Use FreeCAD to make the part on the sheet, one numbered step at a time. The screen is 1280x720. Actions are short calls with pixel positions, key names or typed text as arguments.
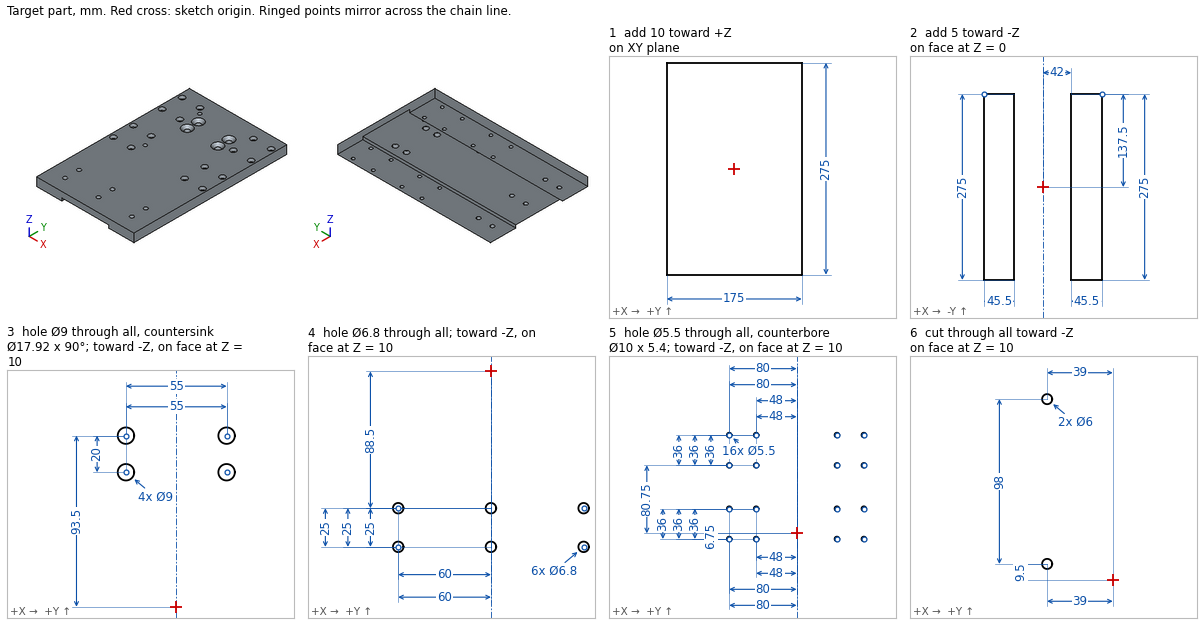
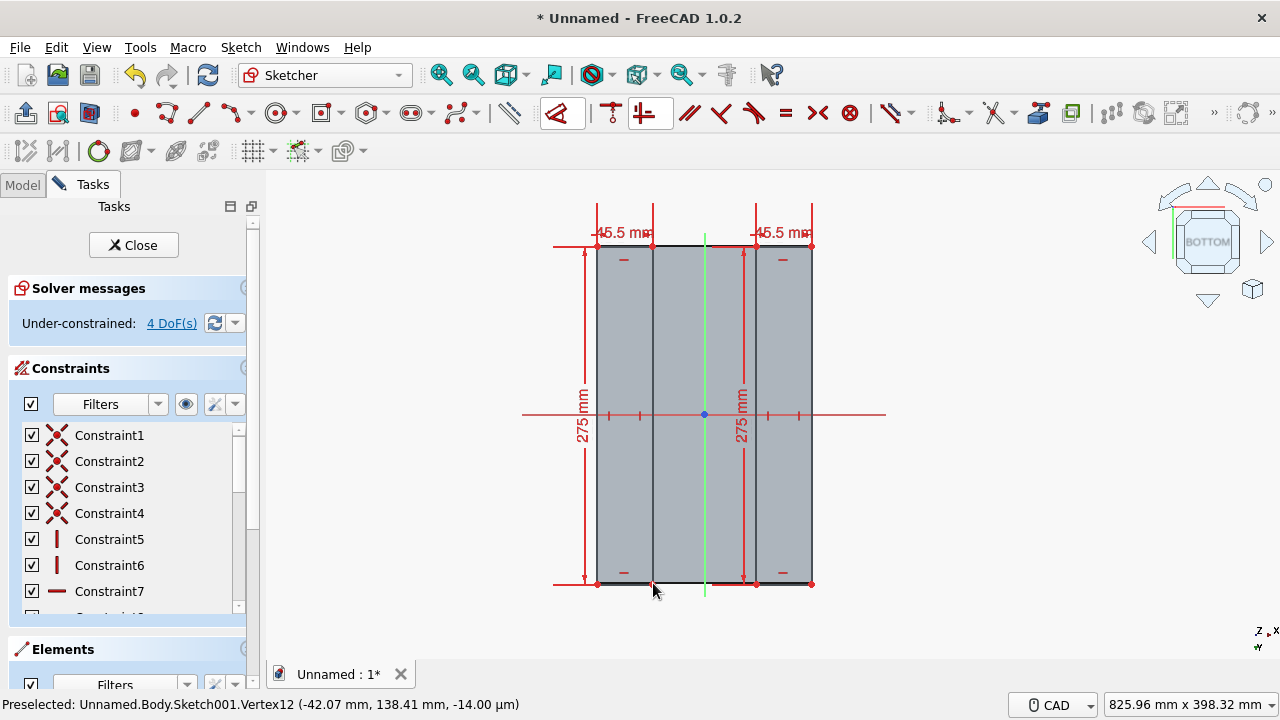
click(812, 247)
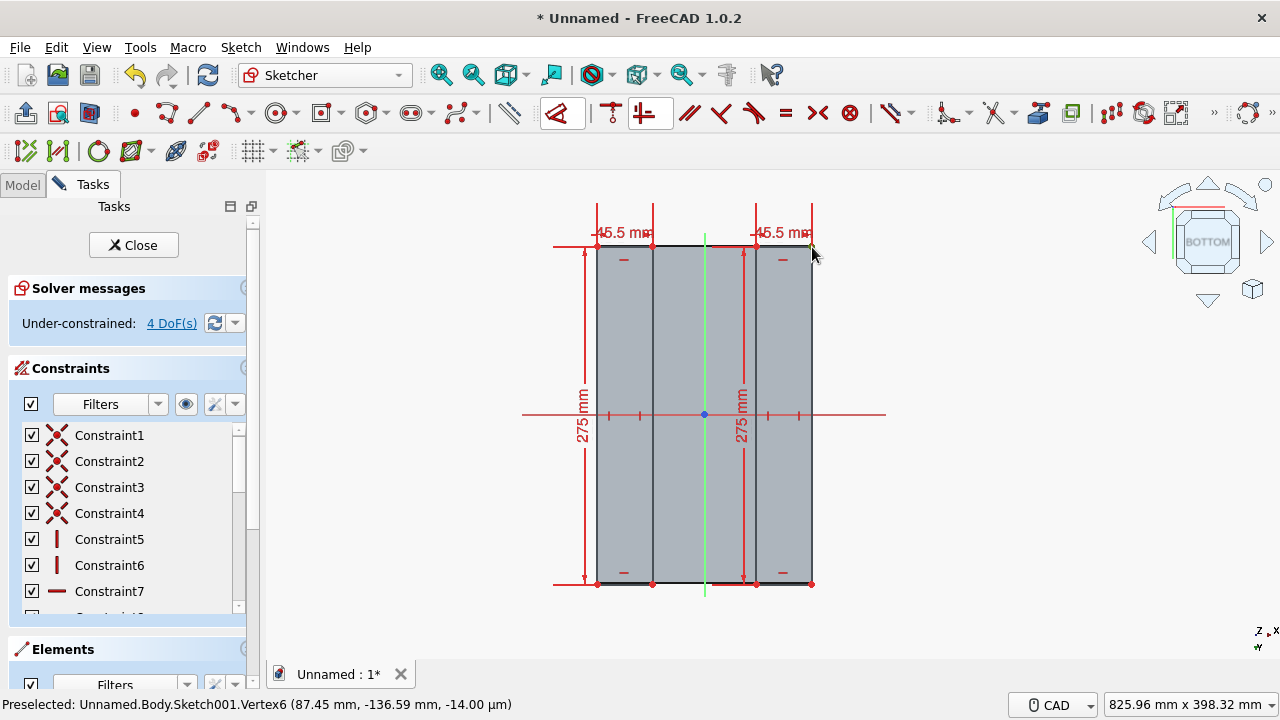
click(597, 247)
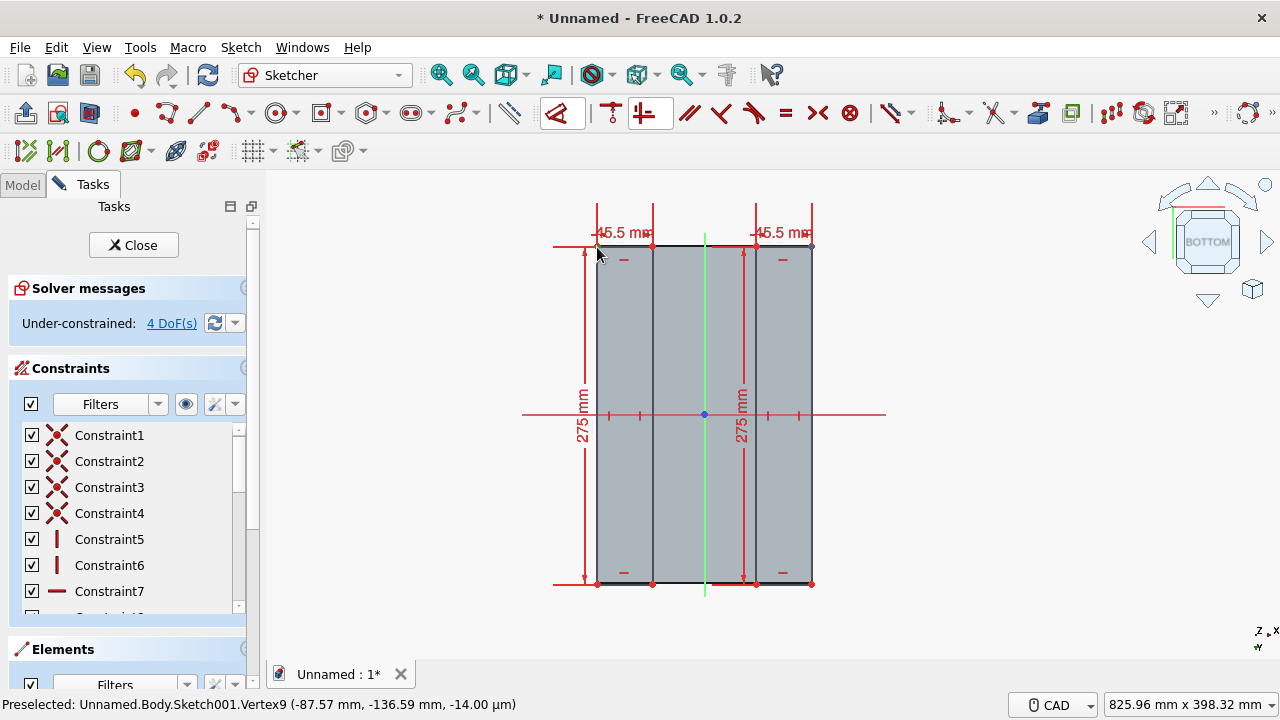
click(705, 600)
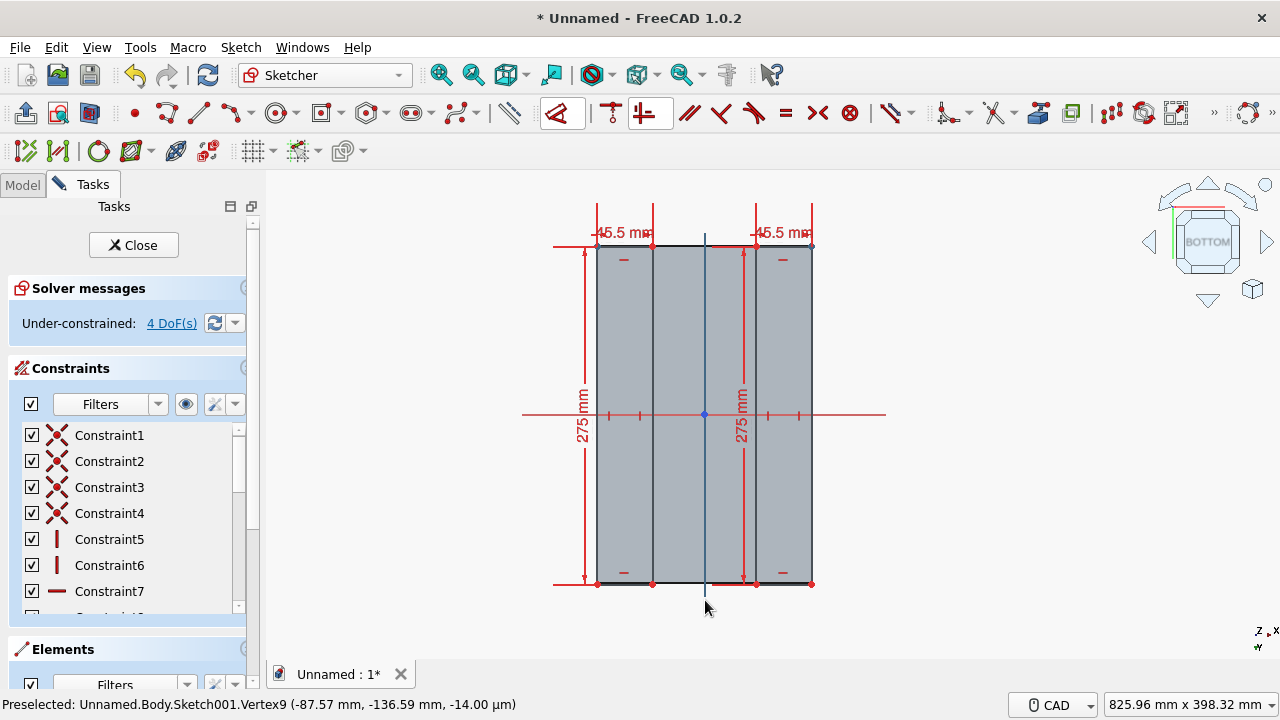
key(s)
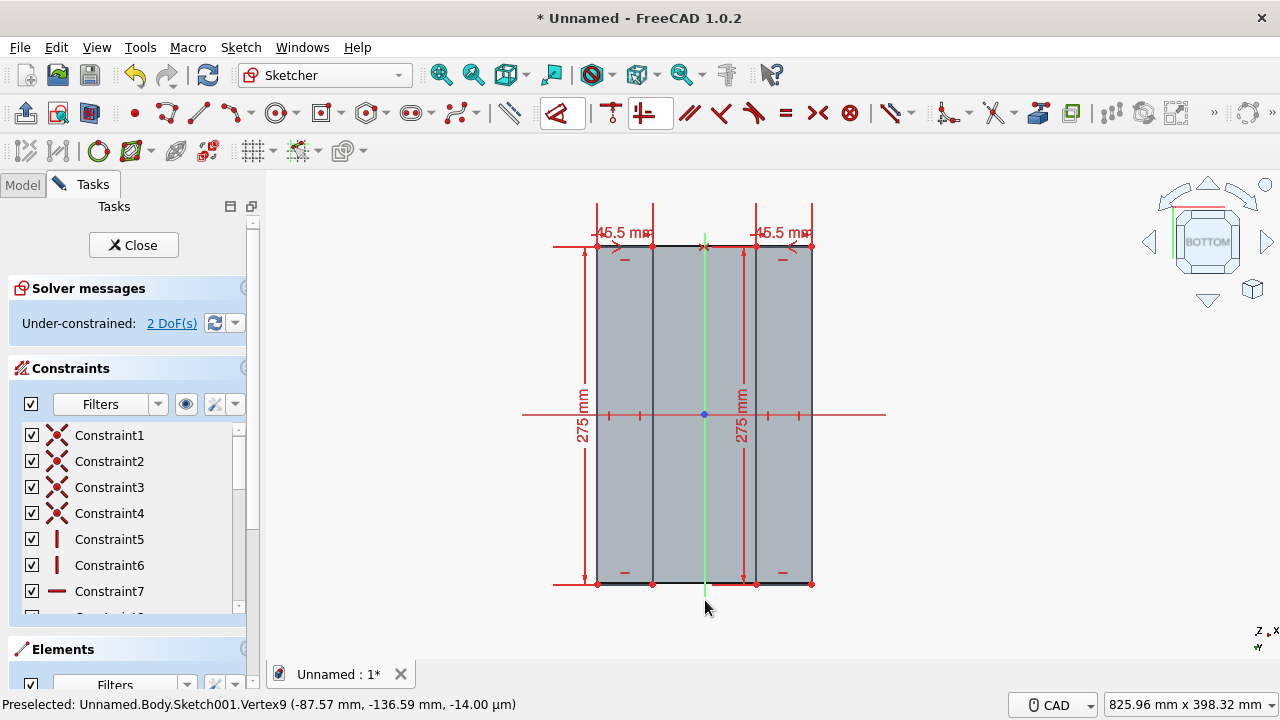
click(556, 114)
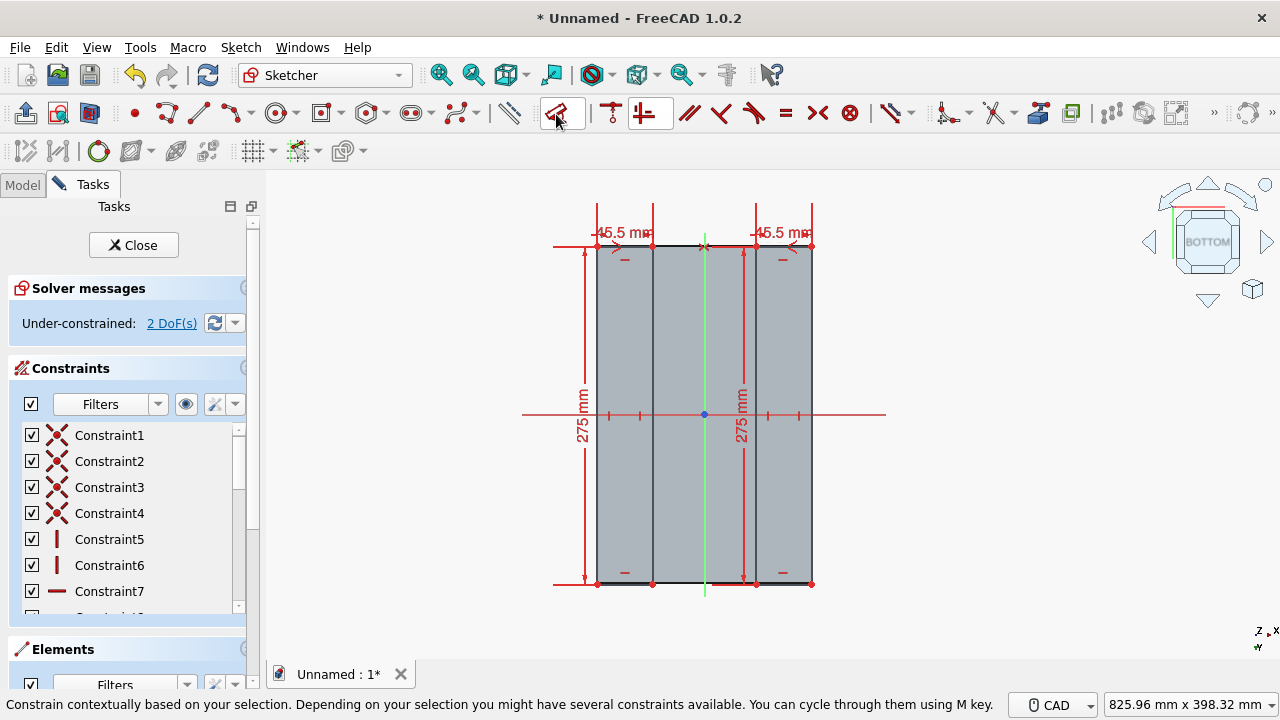
click(756, 247)
click(730, 213)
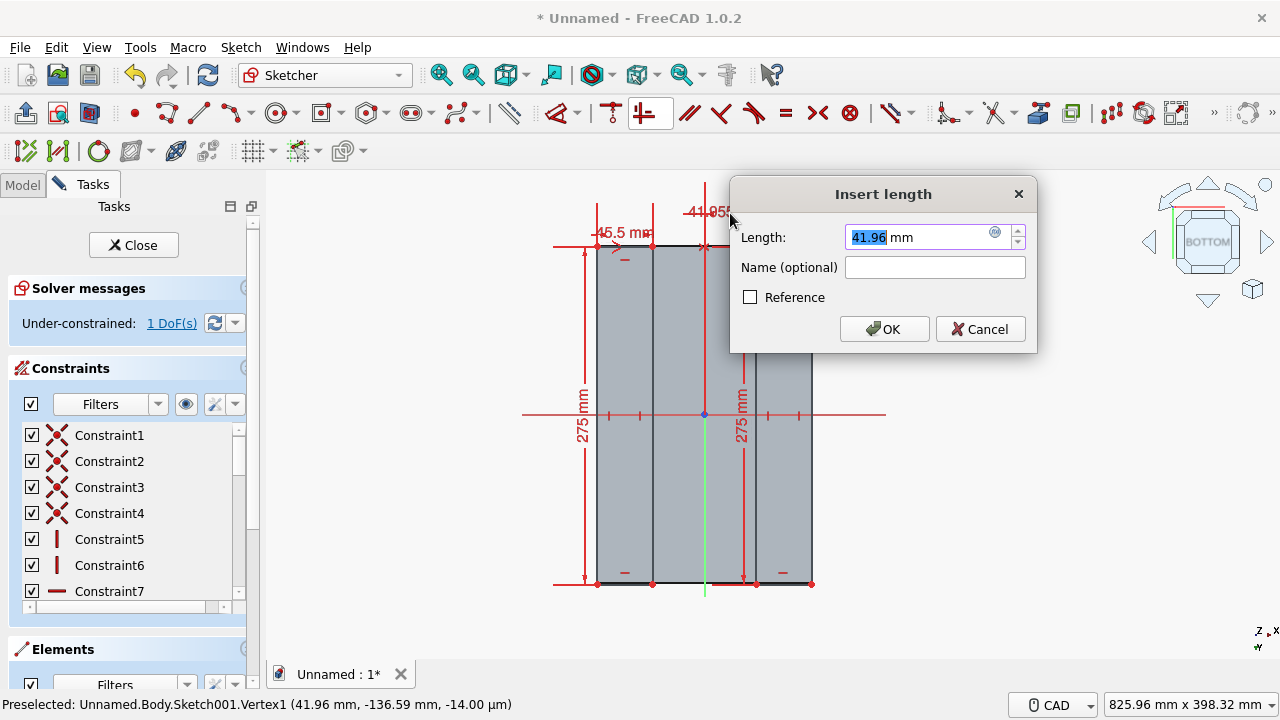
text(42)
key(Return)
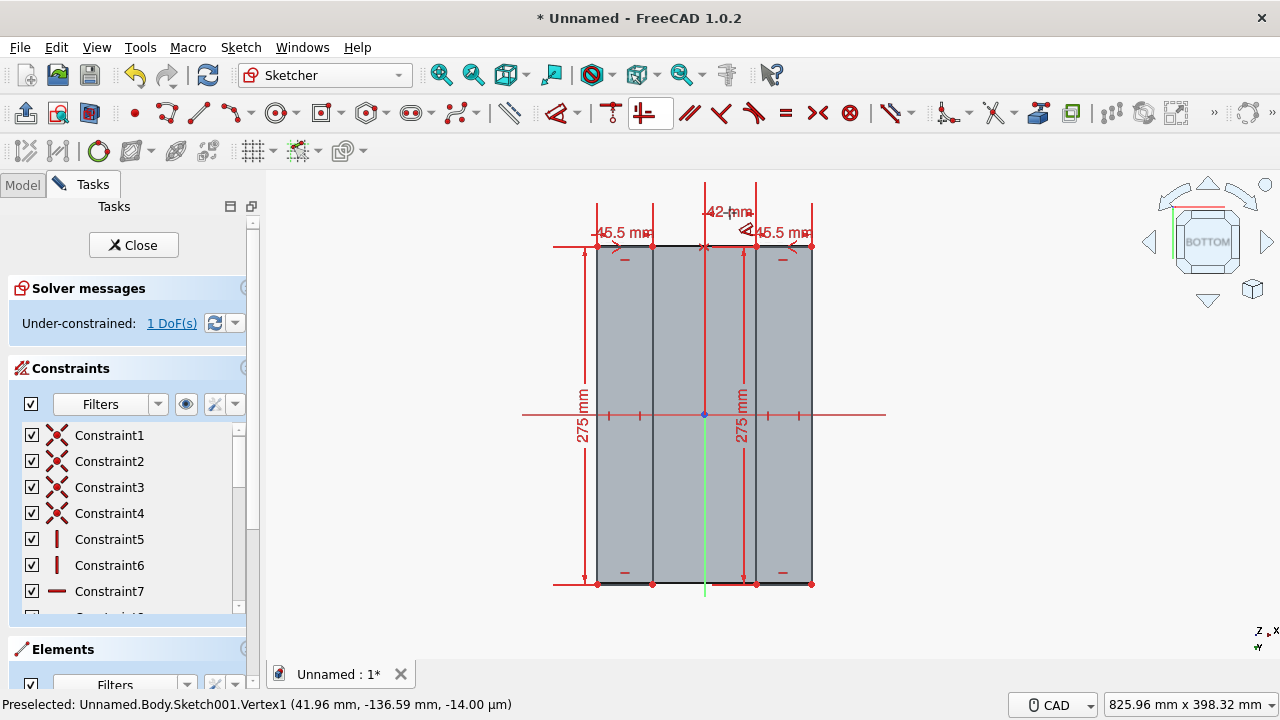
click(756, 247)
click(790, 331)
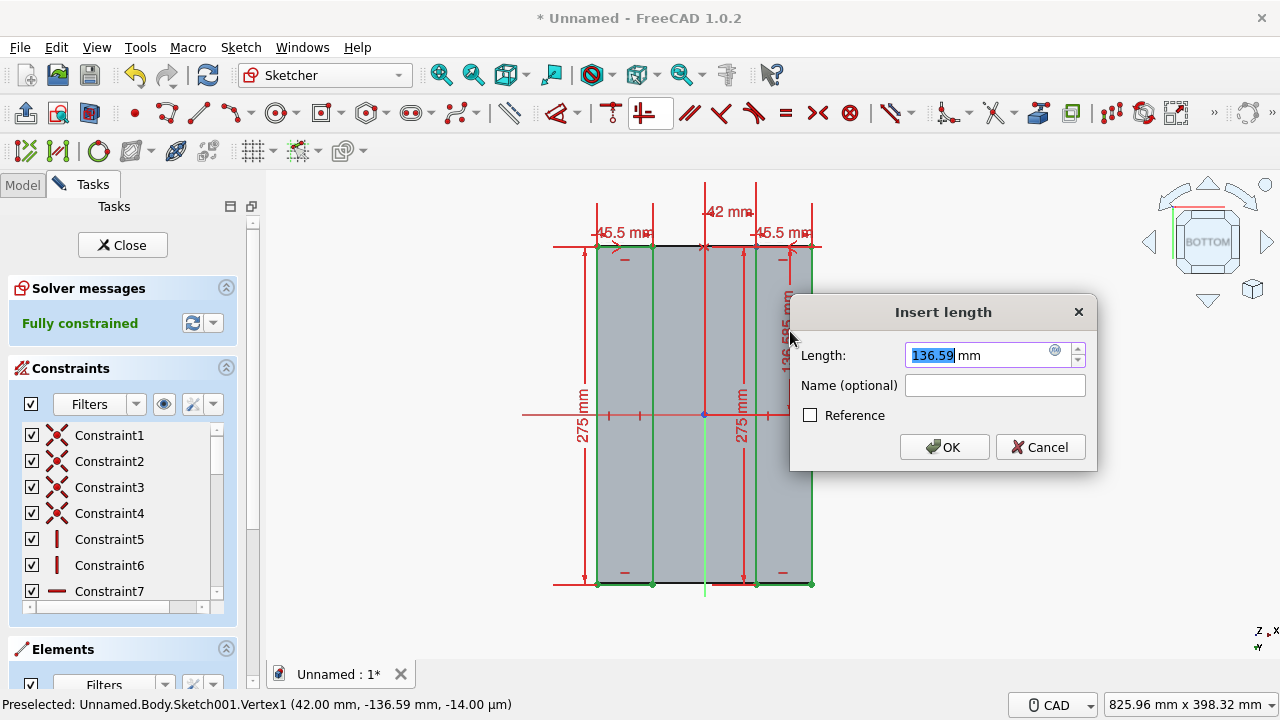
text(137.5)
key(Return)
key(Escape)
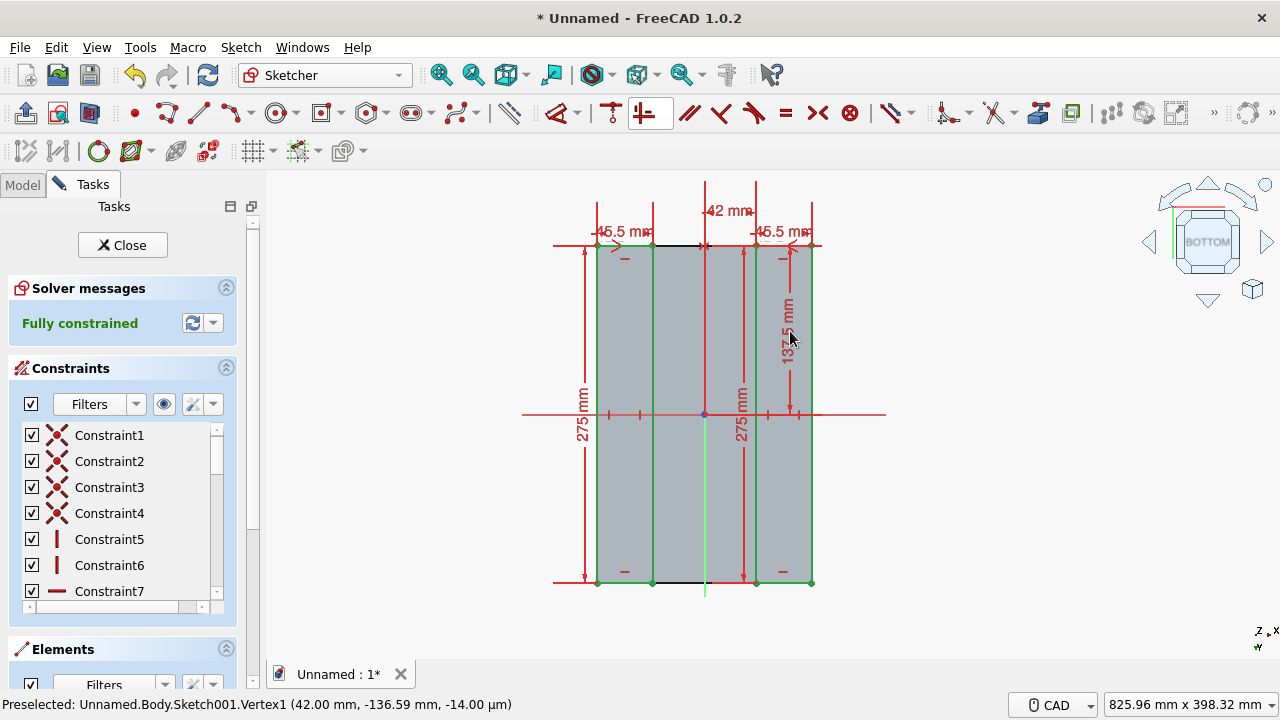
click(123, 245)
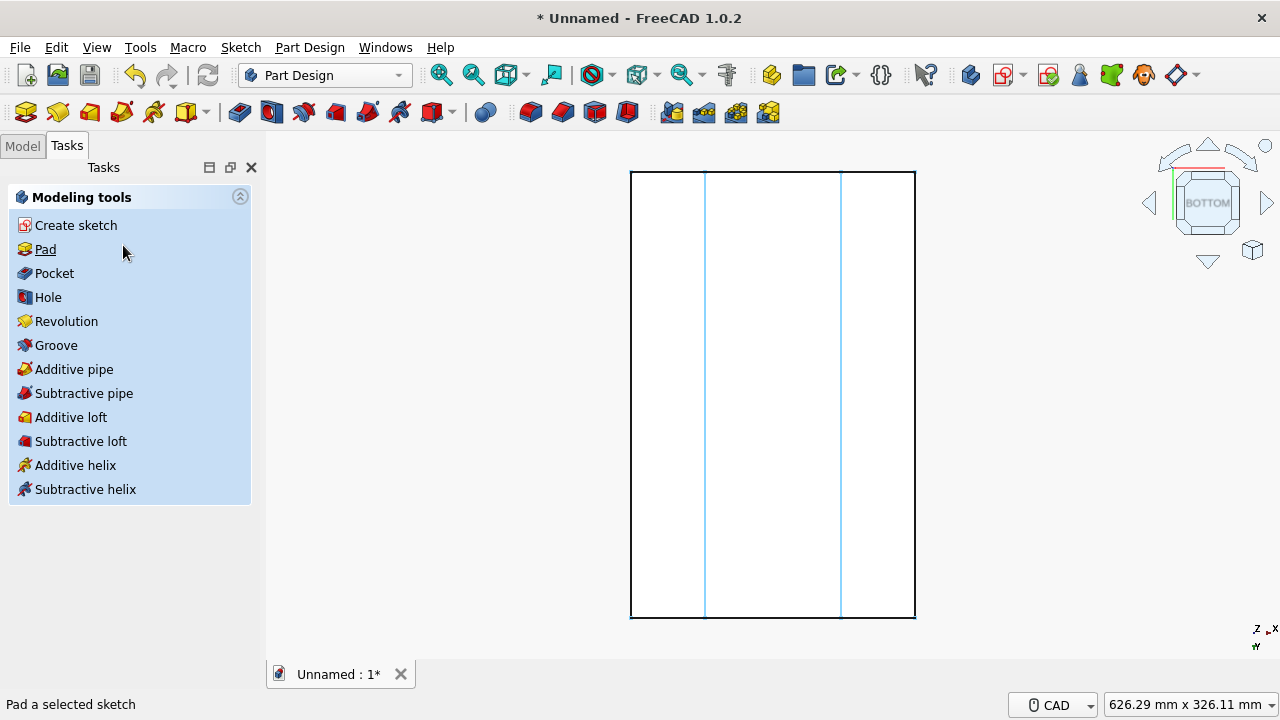
click(26, 112)